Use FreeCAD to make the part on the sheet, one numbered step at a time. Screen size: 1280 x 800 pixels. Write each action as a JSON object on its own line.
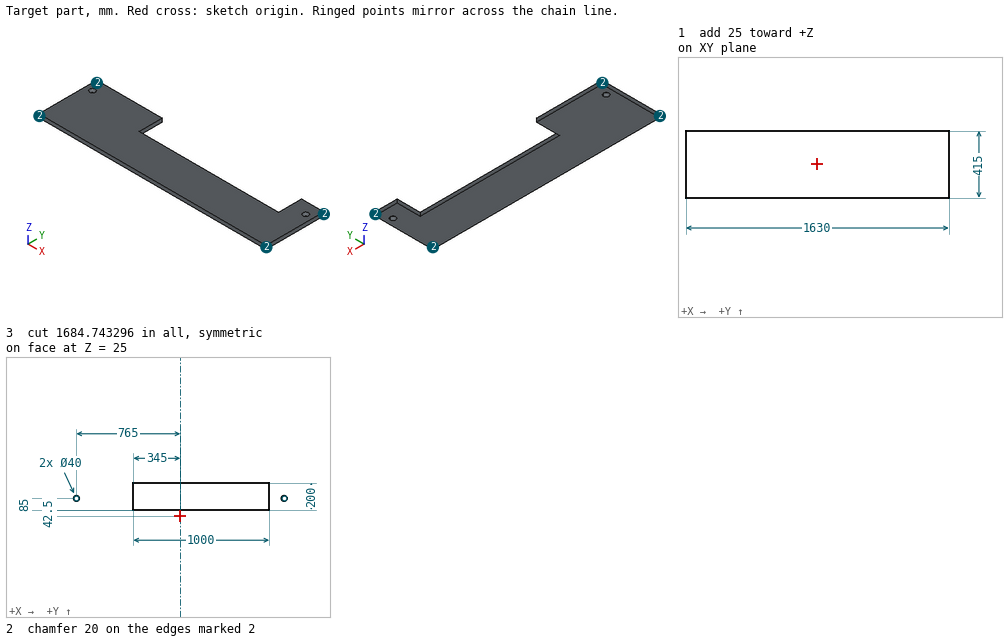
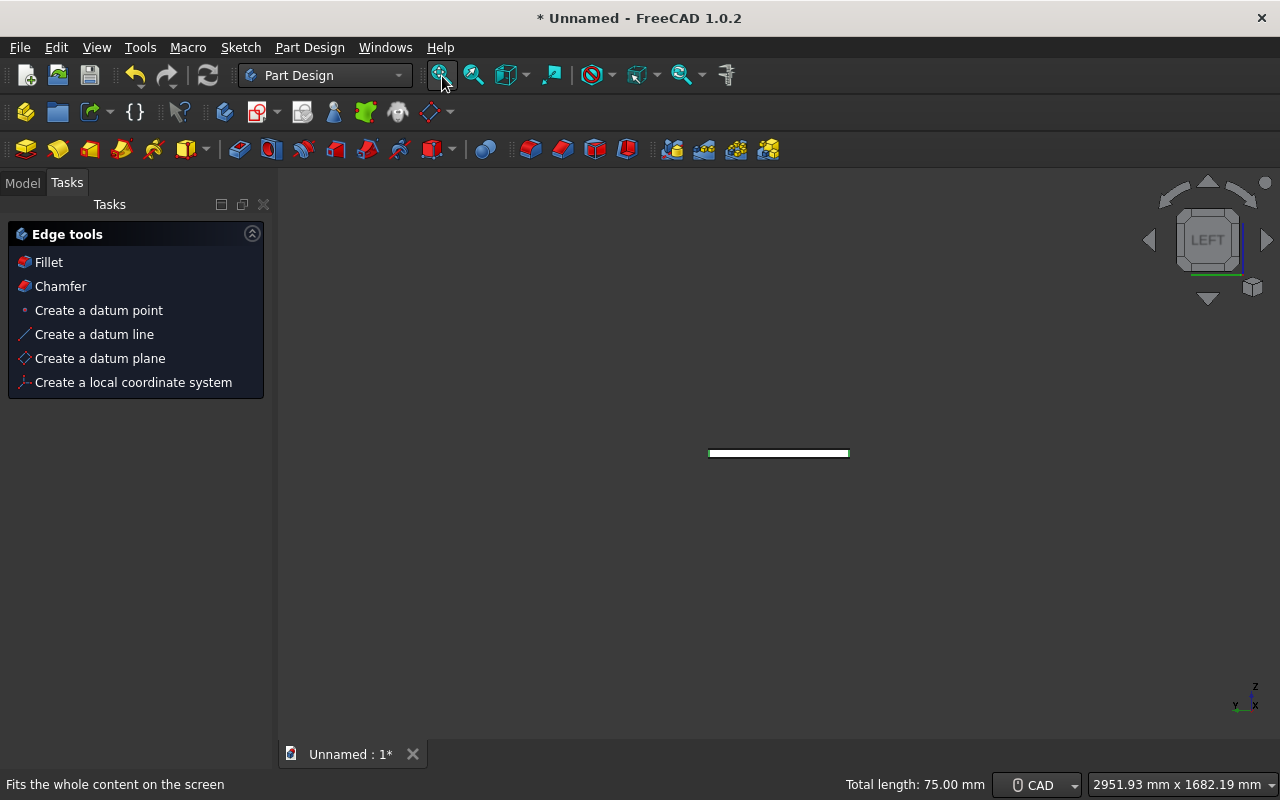
{"action": "scroll", "coordinate": [849, 452], "scroll_direction": "up", "scroll_amount": 8}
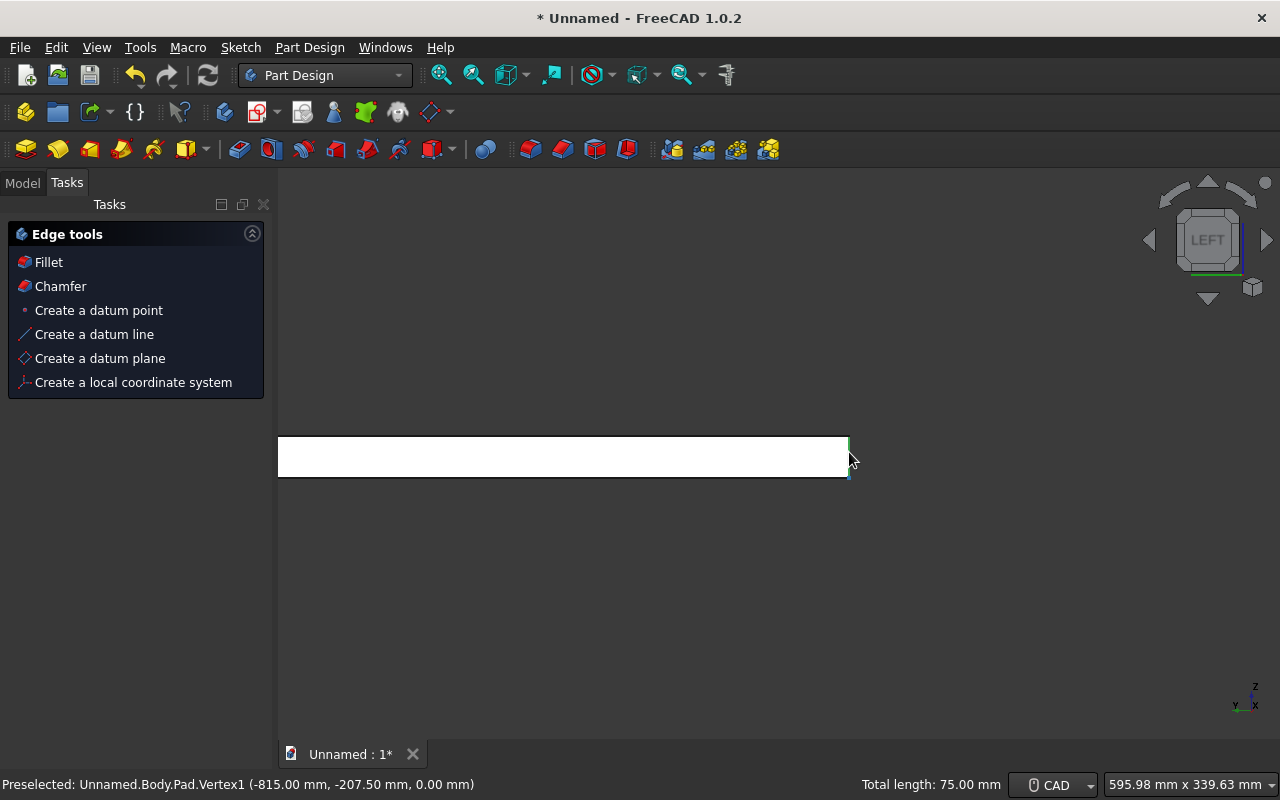
{"action": "left_click", "coordinate": [442, 76]}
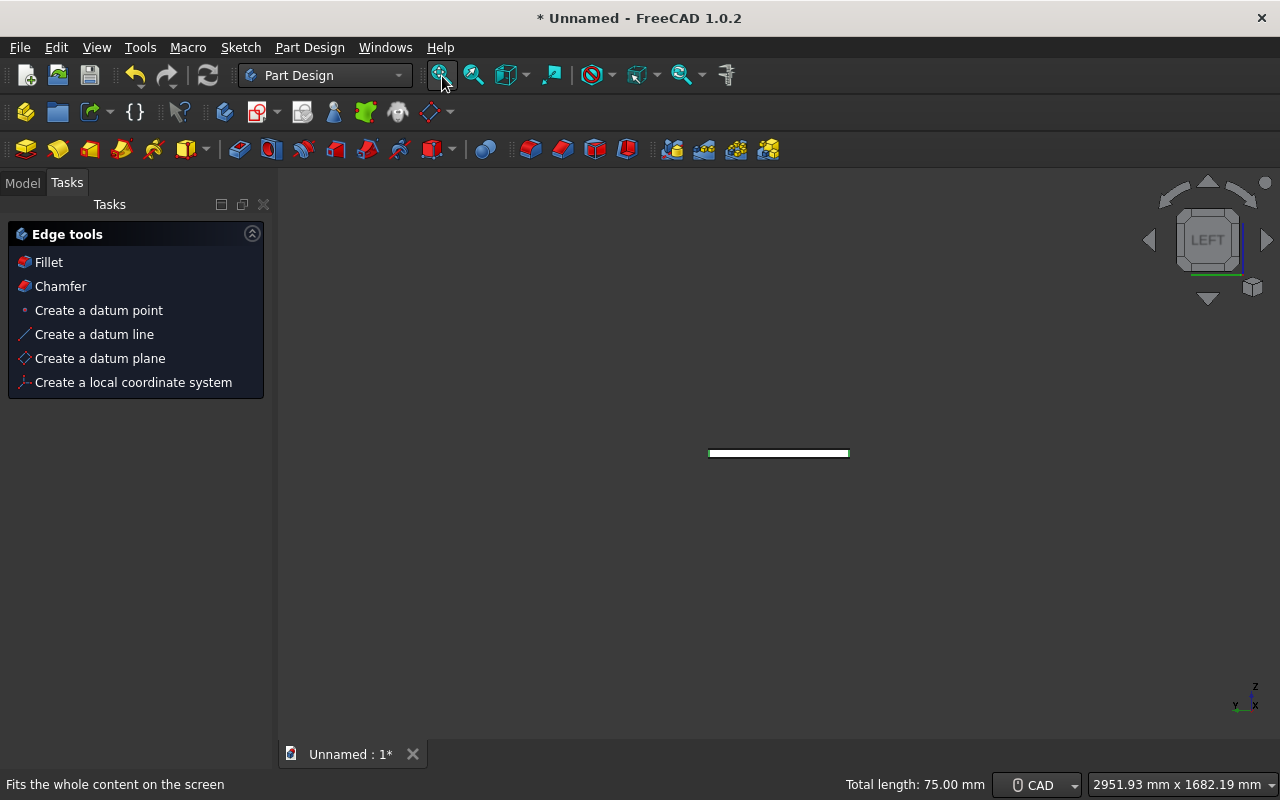
{"action": "key", "text": "v 3"}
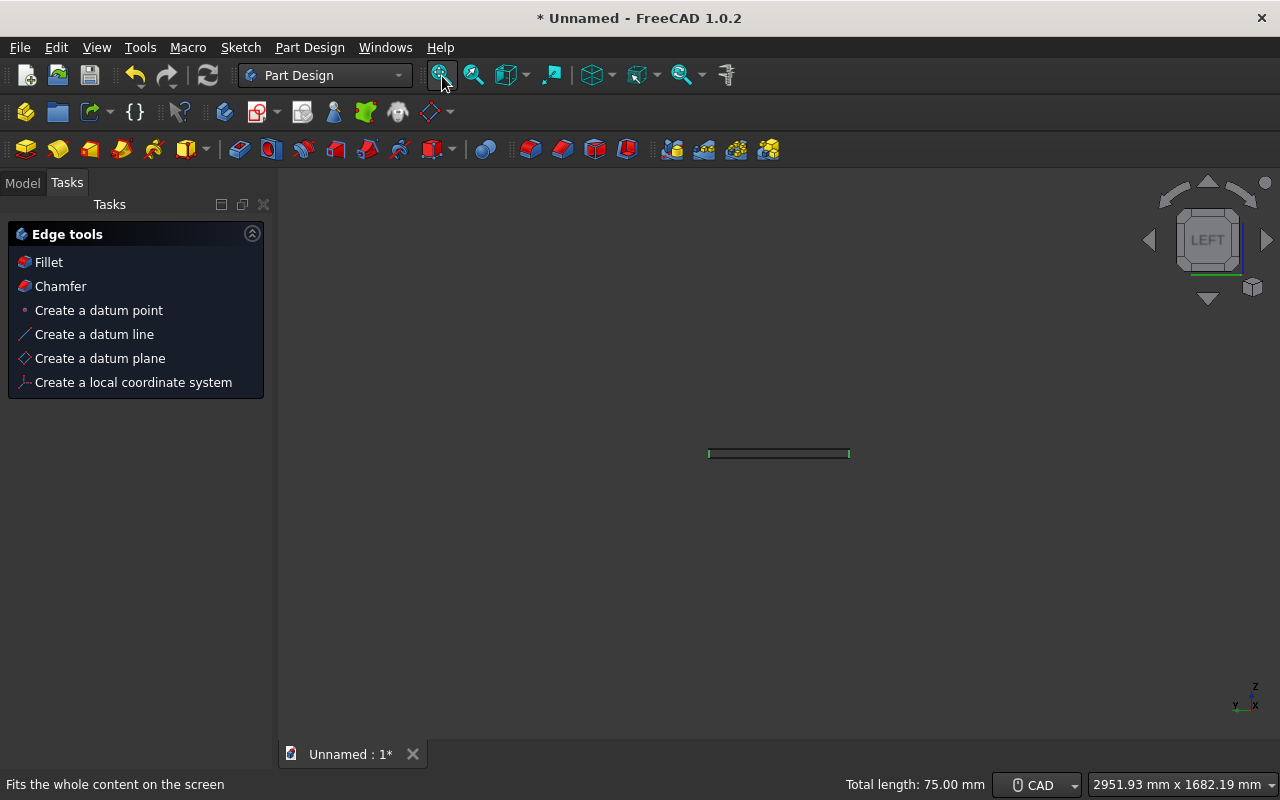
{"action": "key", "text": "0"}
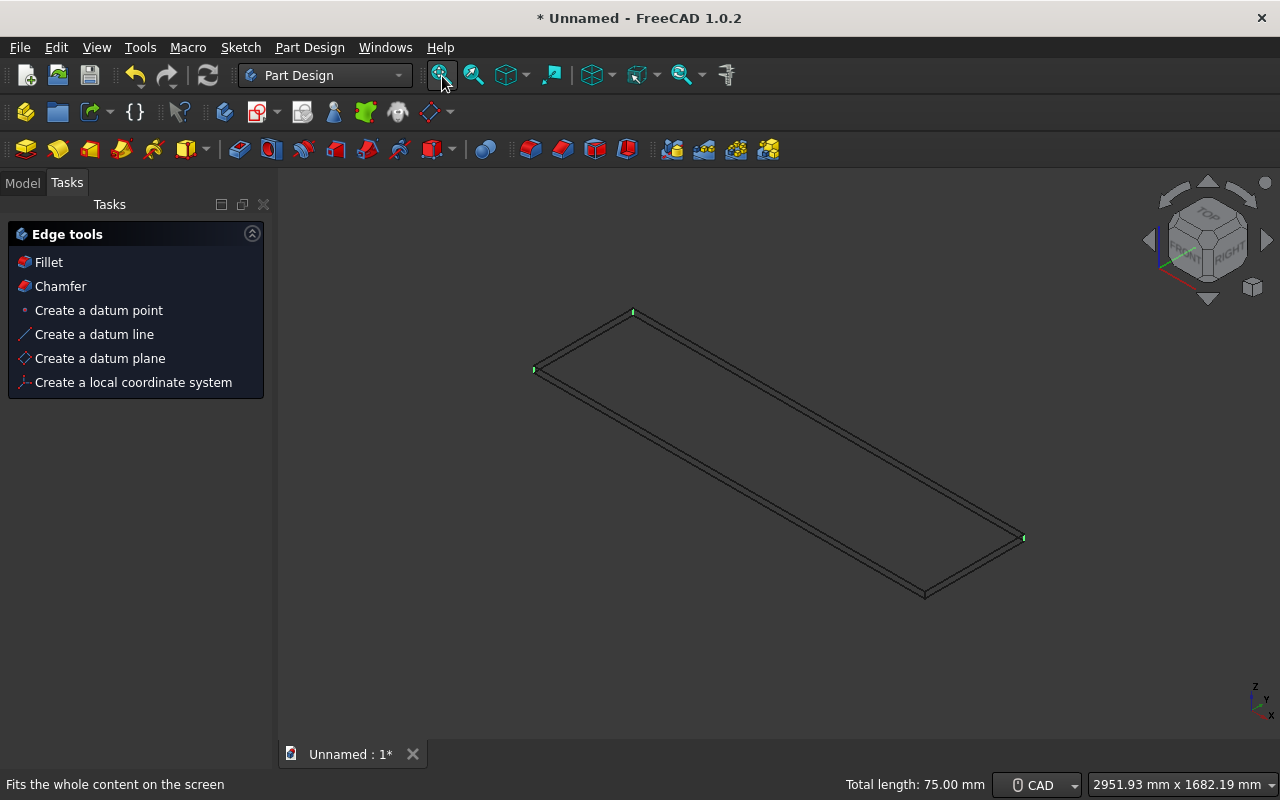
{"action": "left_click", "coordinate": [925, 597], "text": "ctrl"}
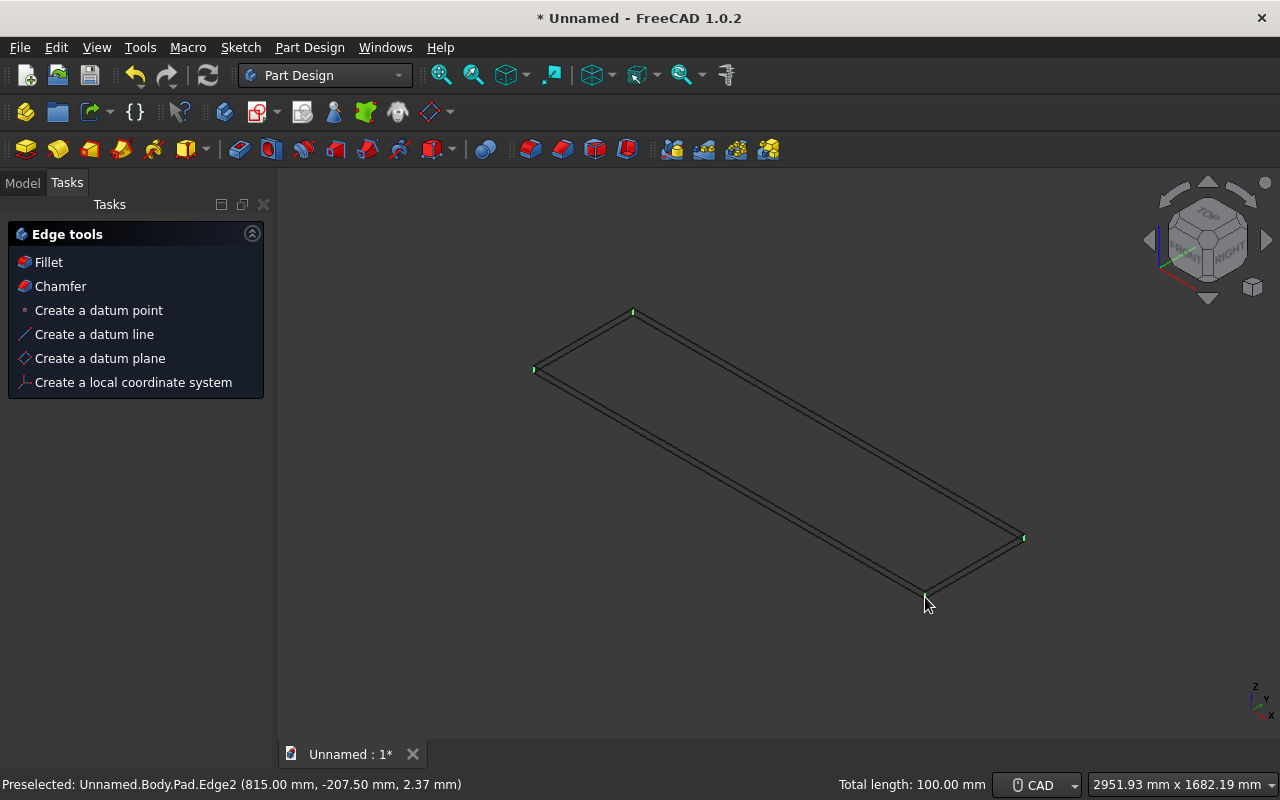
{"action": "key", "text": "v 1"}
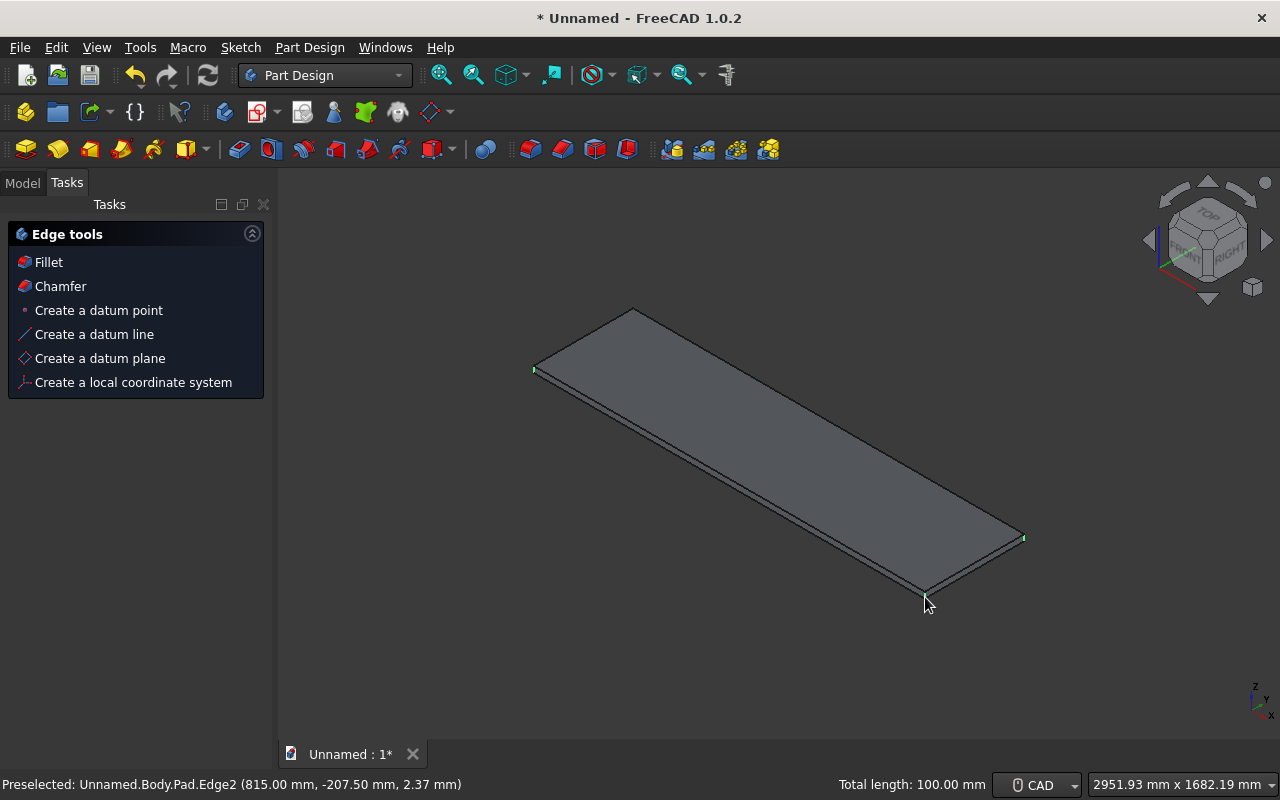
{"action": "left_click", "coordinate": [564, 150]}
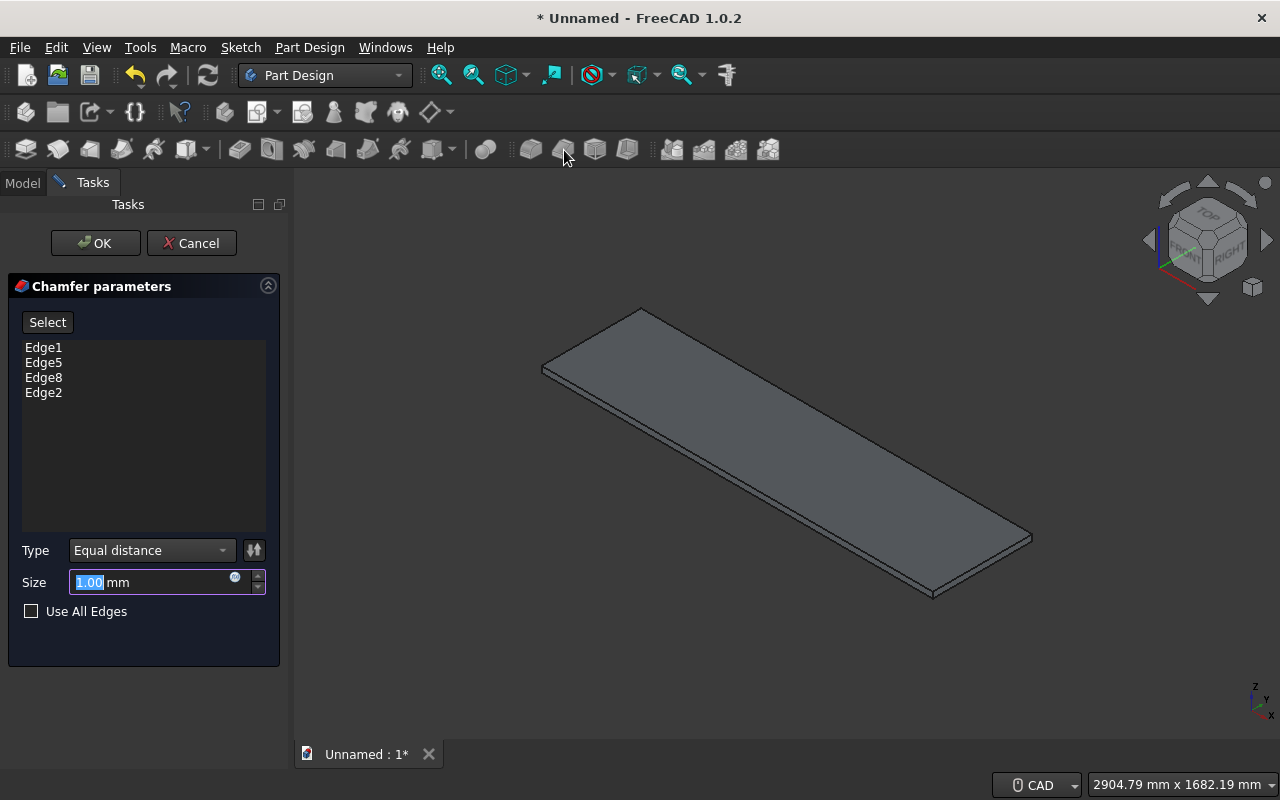
{"action": "type", "text": "20"}
{"action": "key", "text": "Tab"}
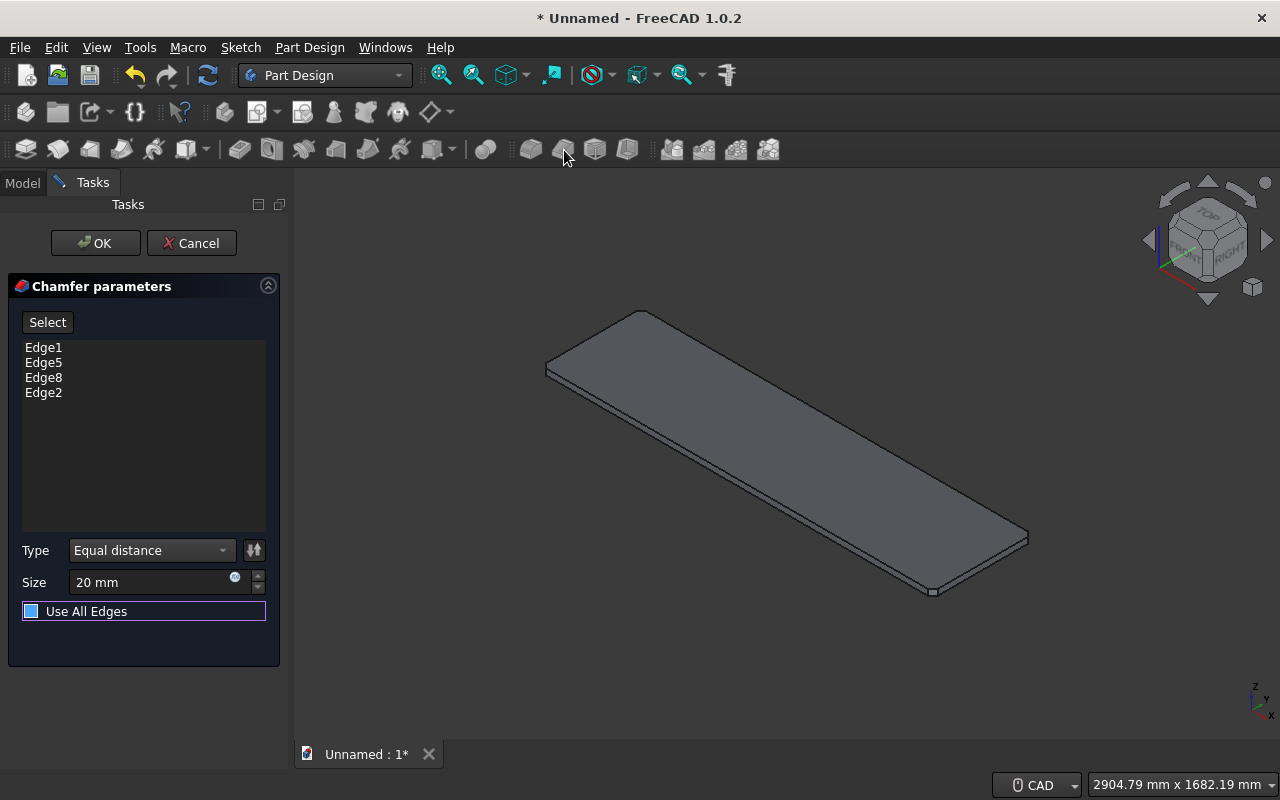
{"action": "left_click", "coordinate": [96, 243]}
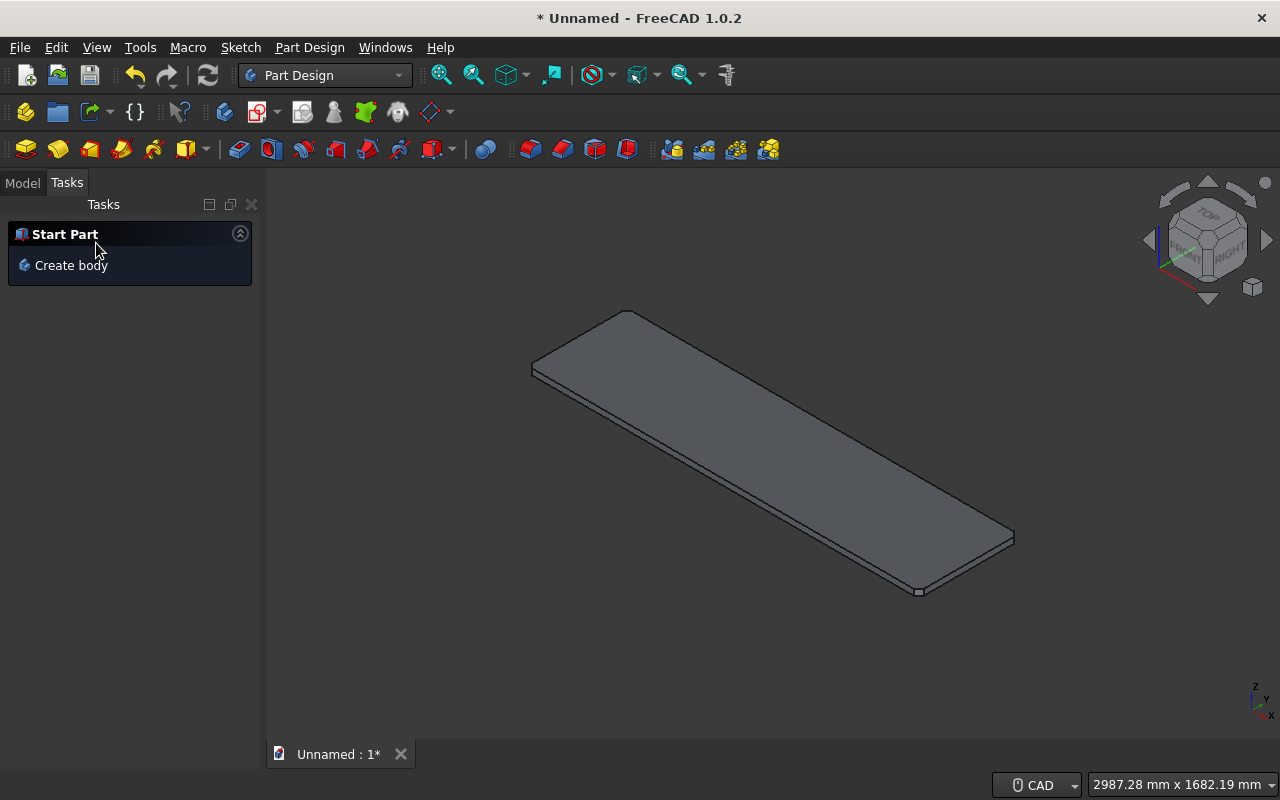
{"action": "left_click", "coordinate": [885, 514]}